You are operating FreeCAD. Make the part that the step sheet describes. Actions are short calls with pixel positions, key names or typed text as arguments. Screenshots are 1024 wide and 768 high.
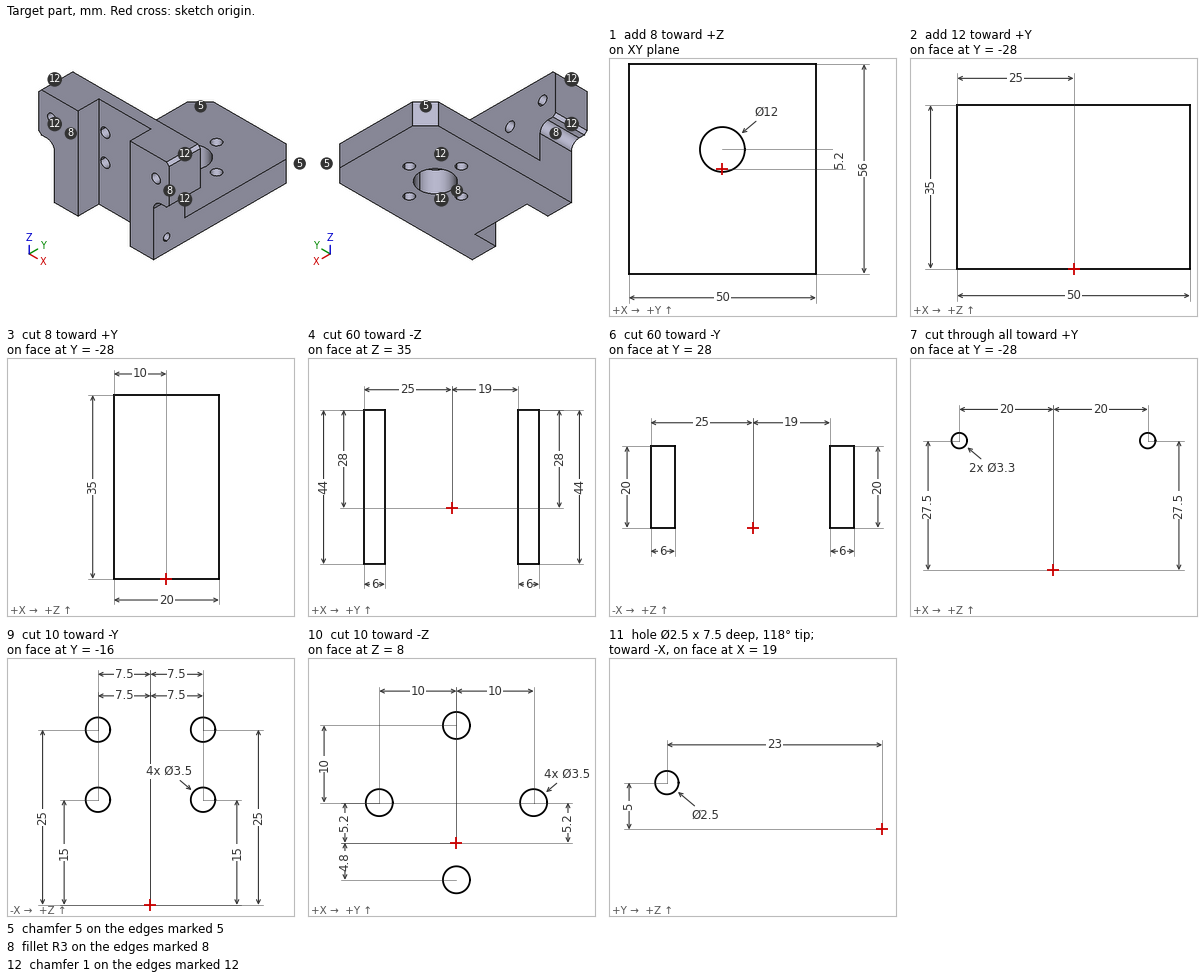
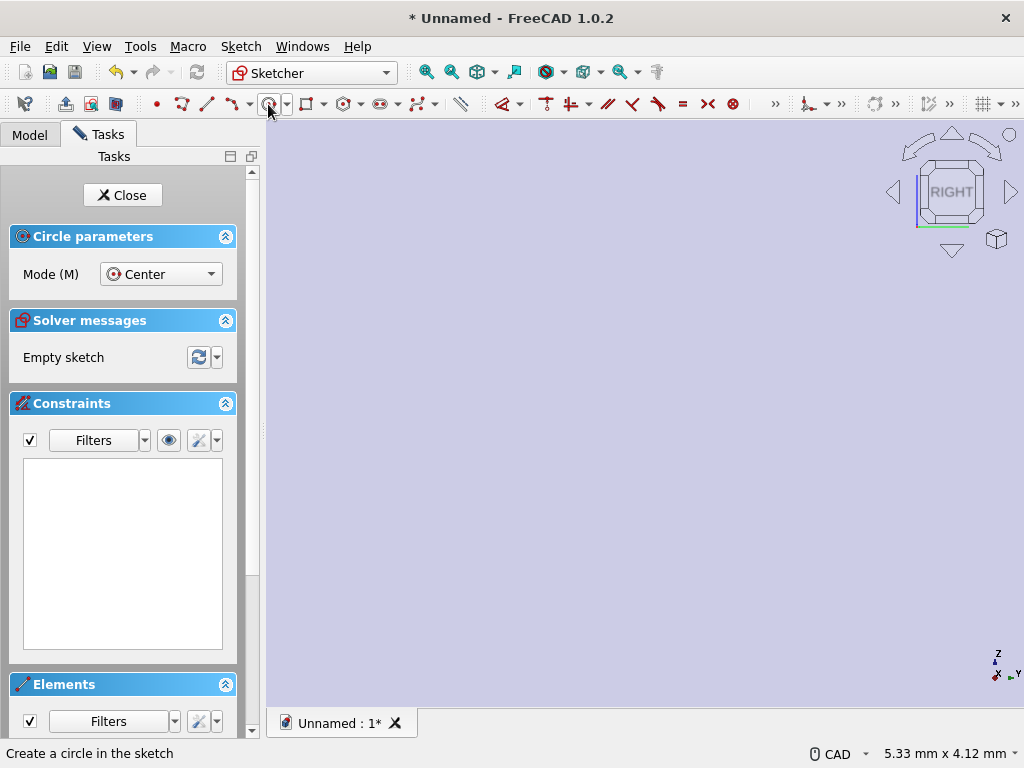
click(572, 396)
move(698, 270)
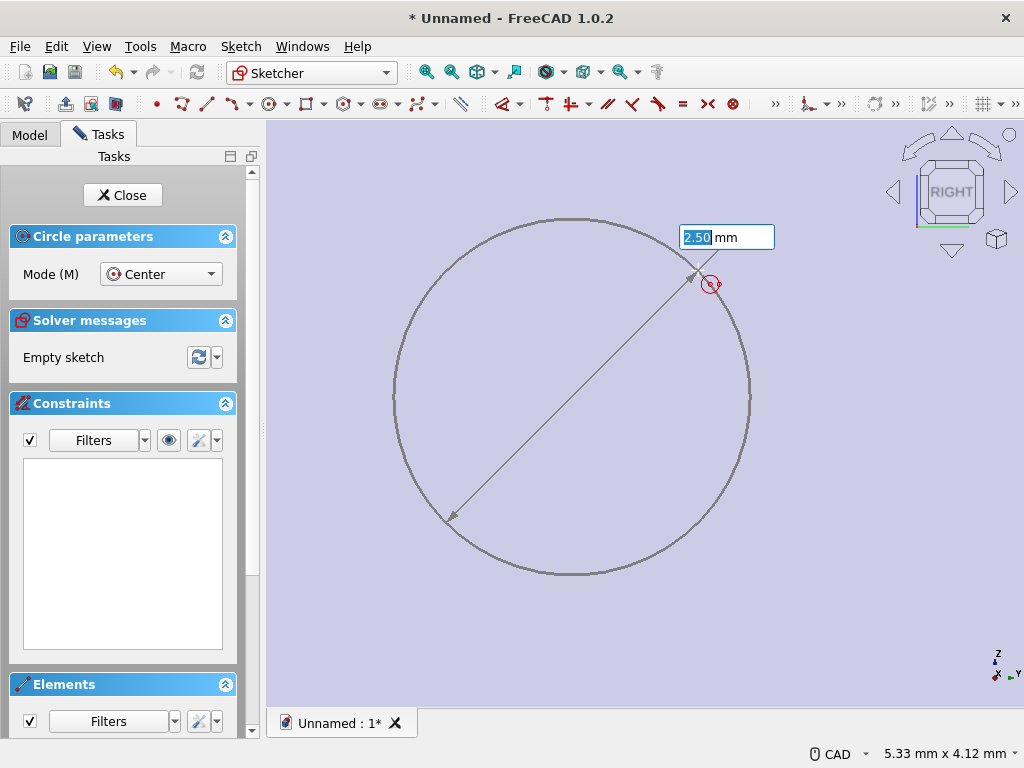
text(2.5)
key(Return)
key(Escape)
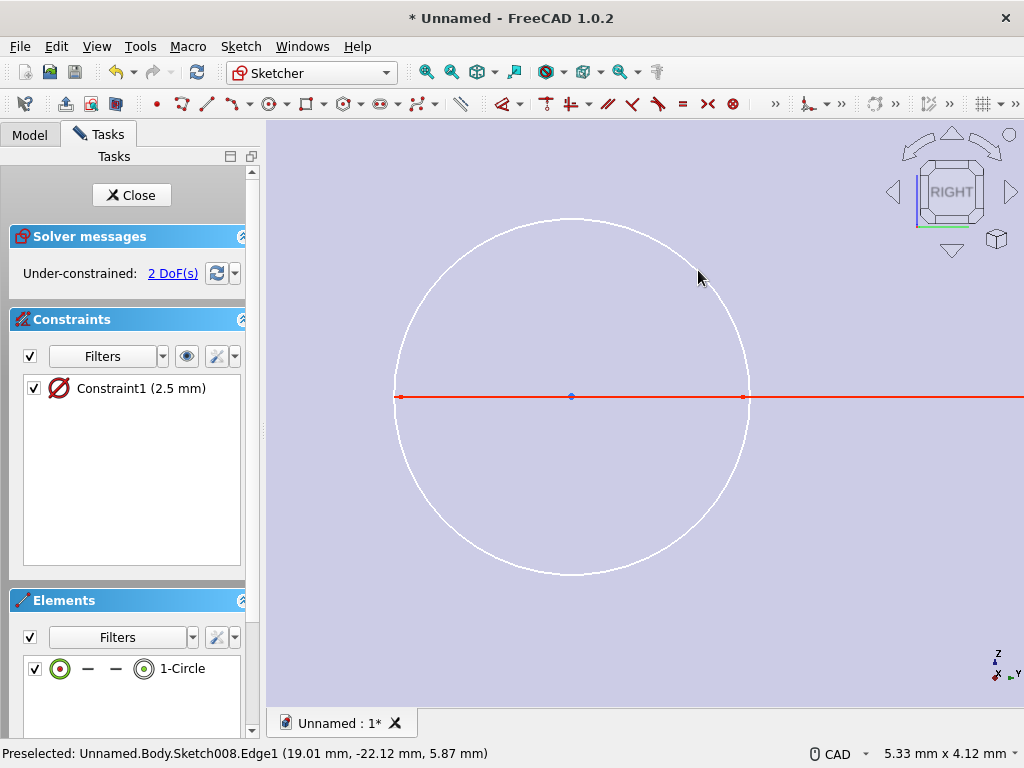
click(502, 104)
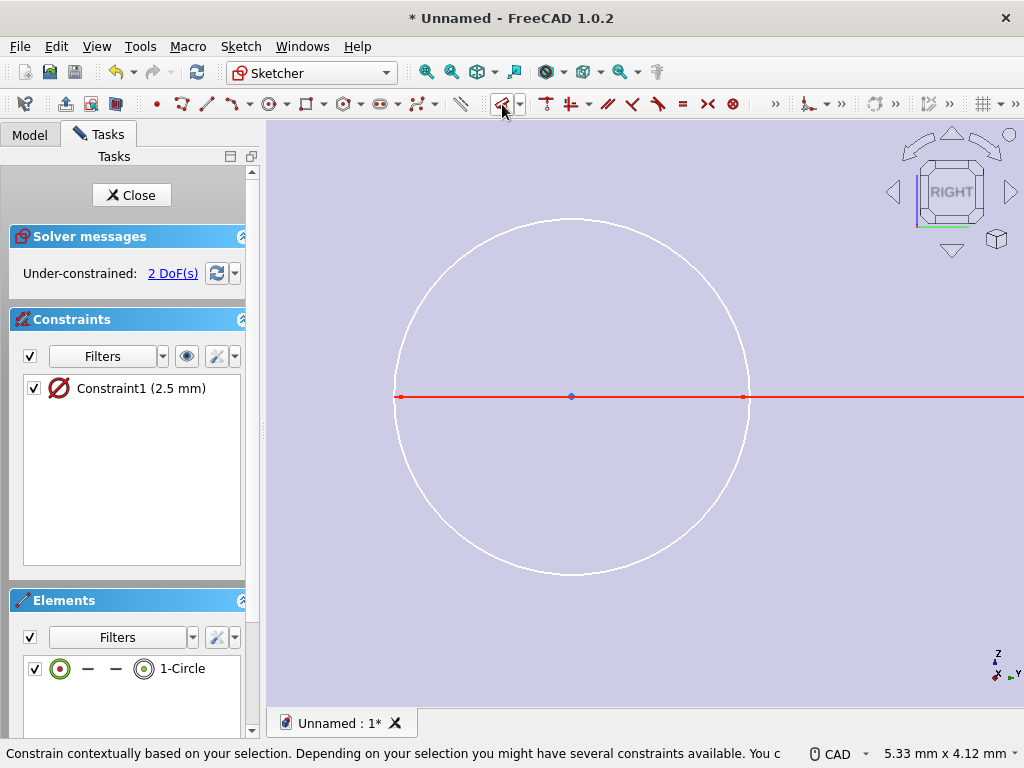
click(572, 397)
click(538, 538)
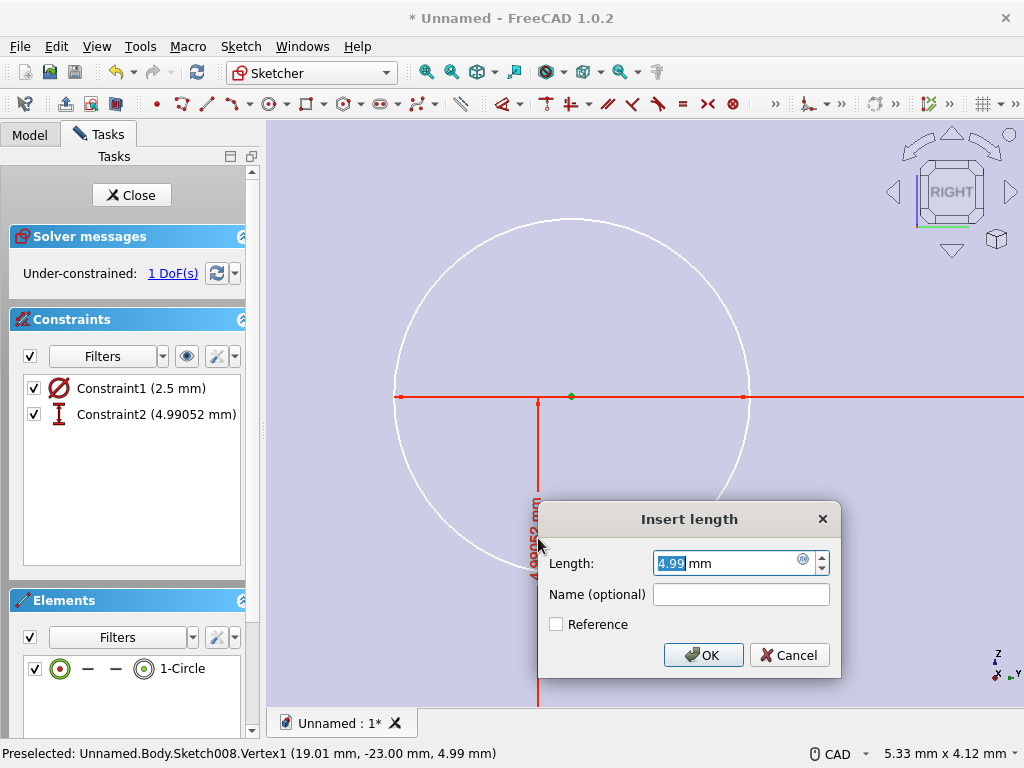
text(5)
key(Return)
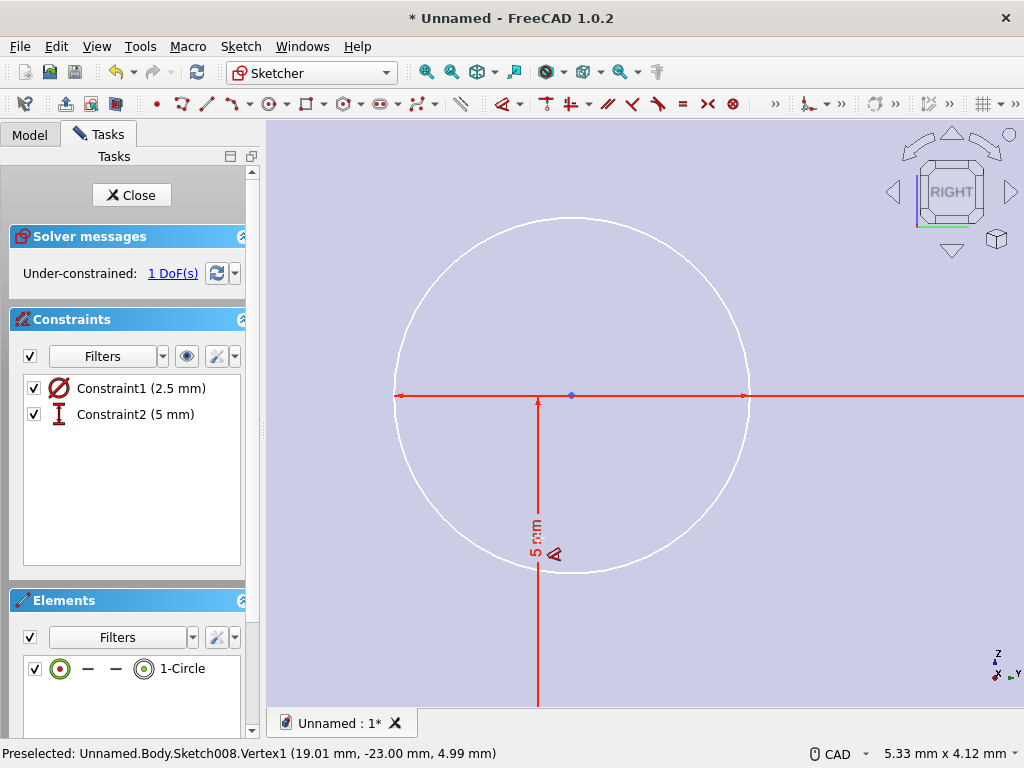
click(572, 396)
click(716, 362)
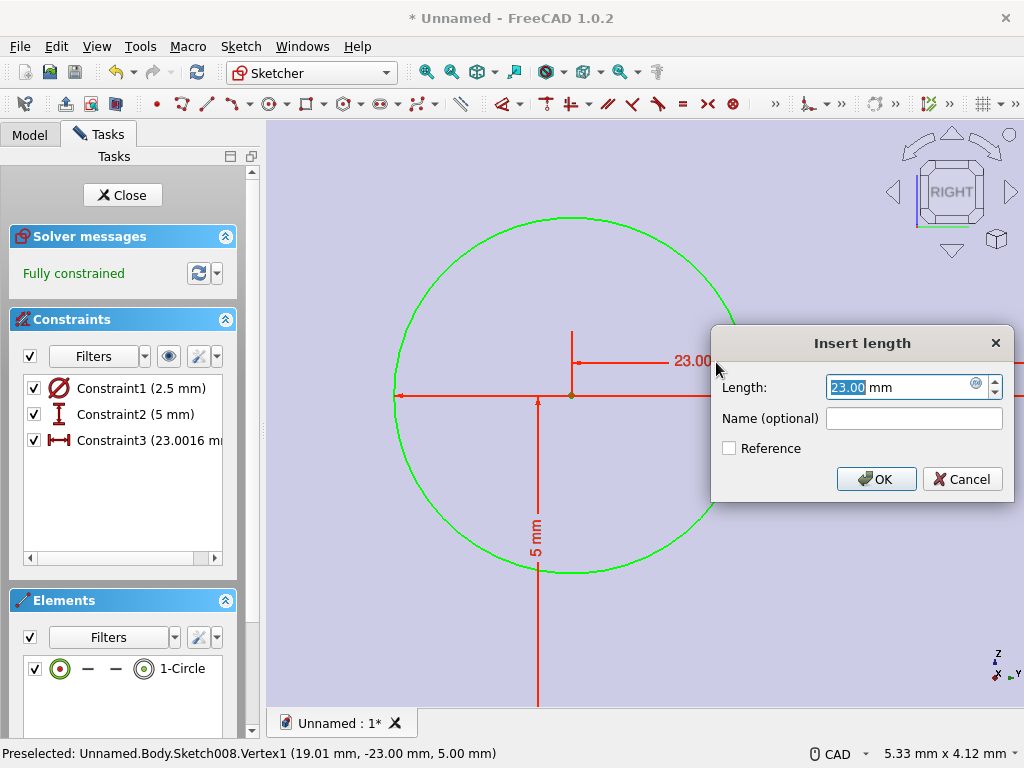
text(23)
key(Return)
key(Escape)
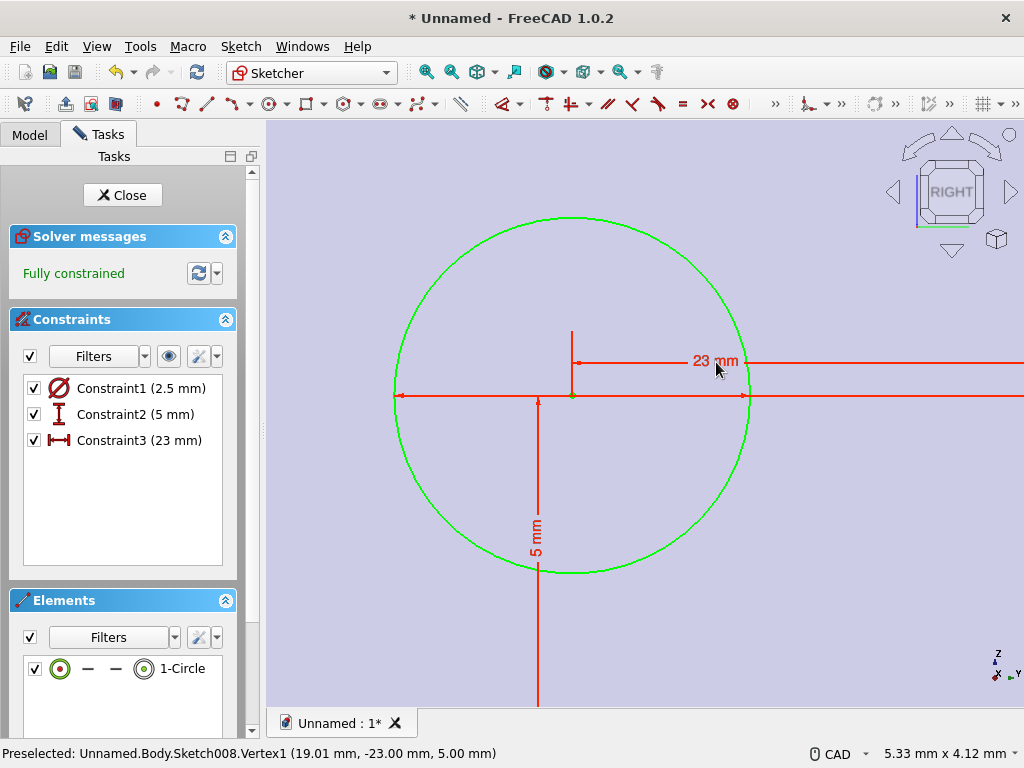
click(123, 195)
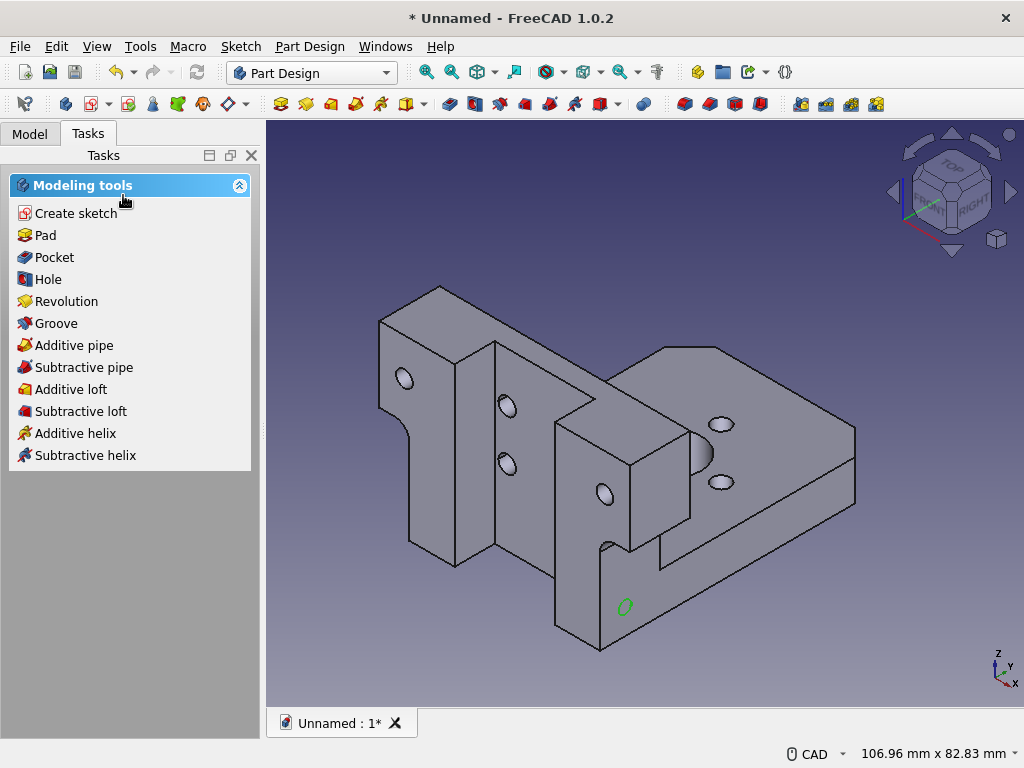
click(475, 104)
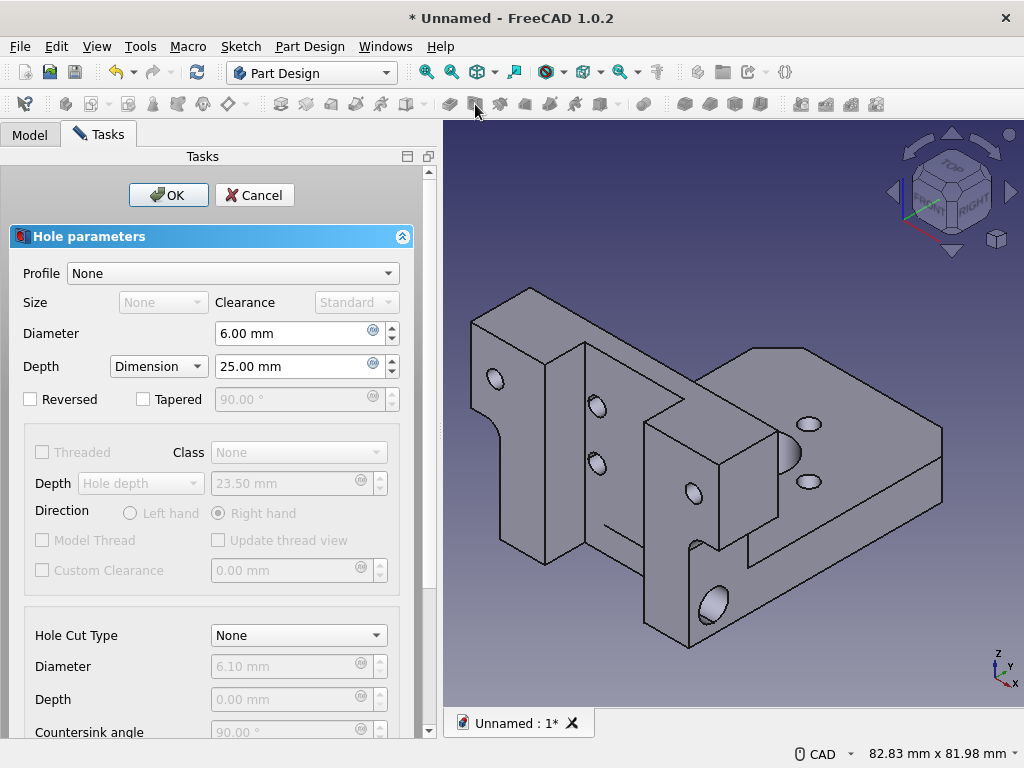
triple_click(300, 334)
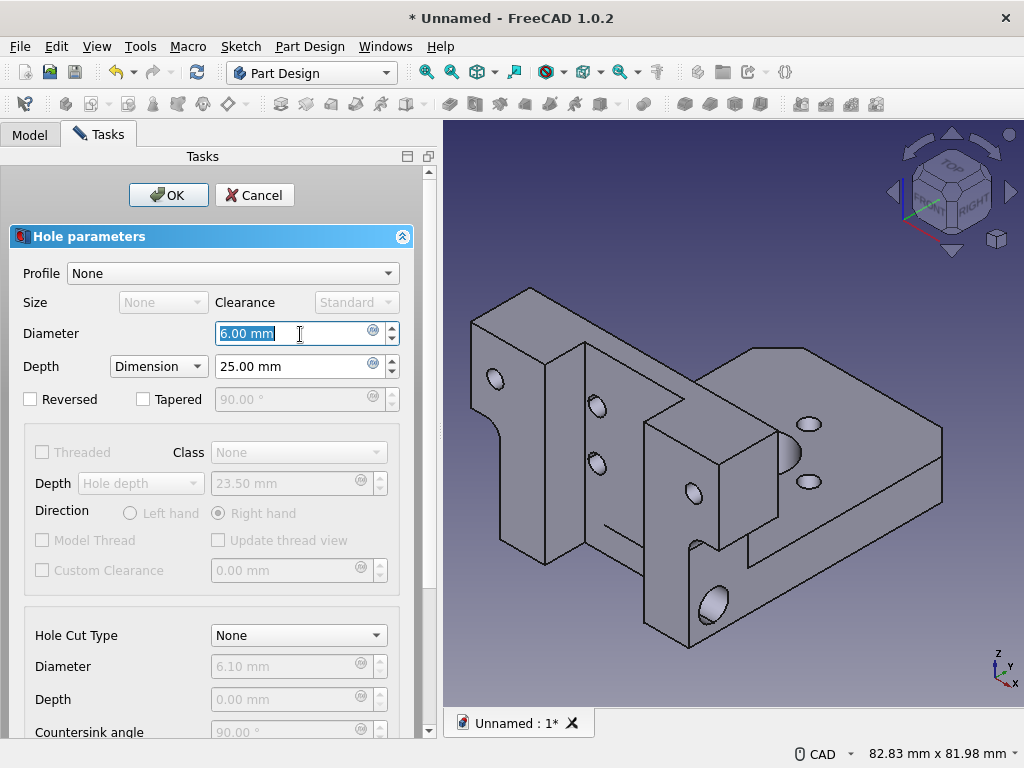
text(2.5)
key(Tab)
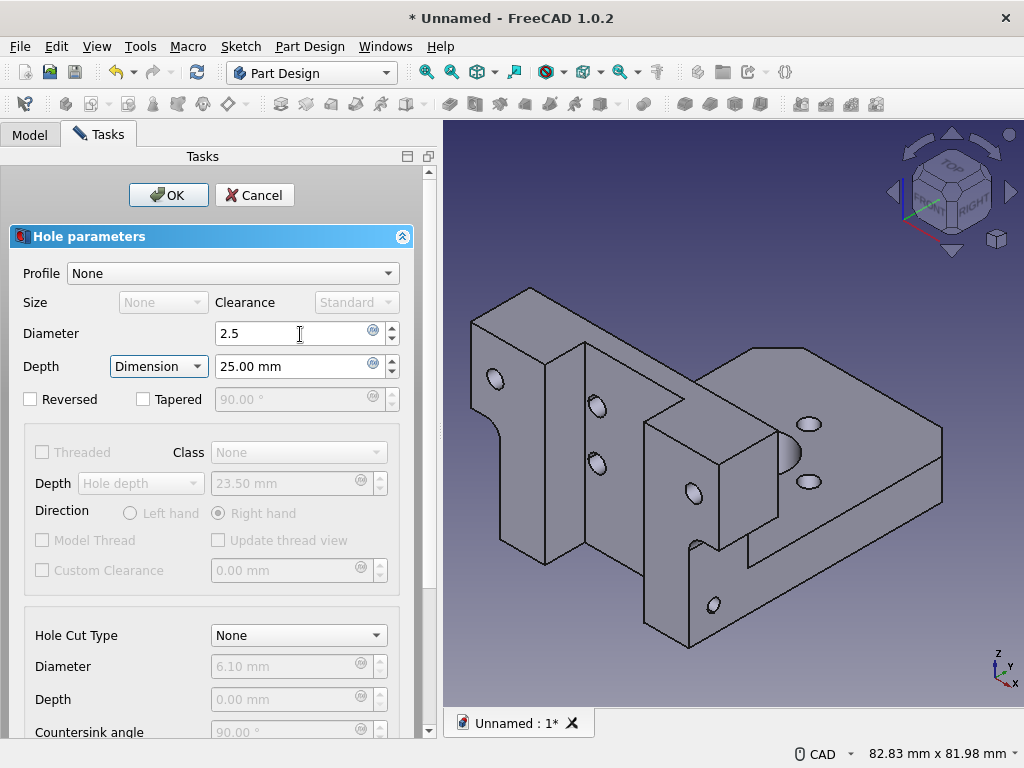
triple_click(300, 366)